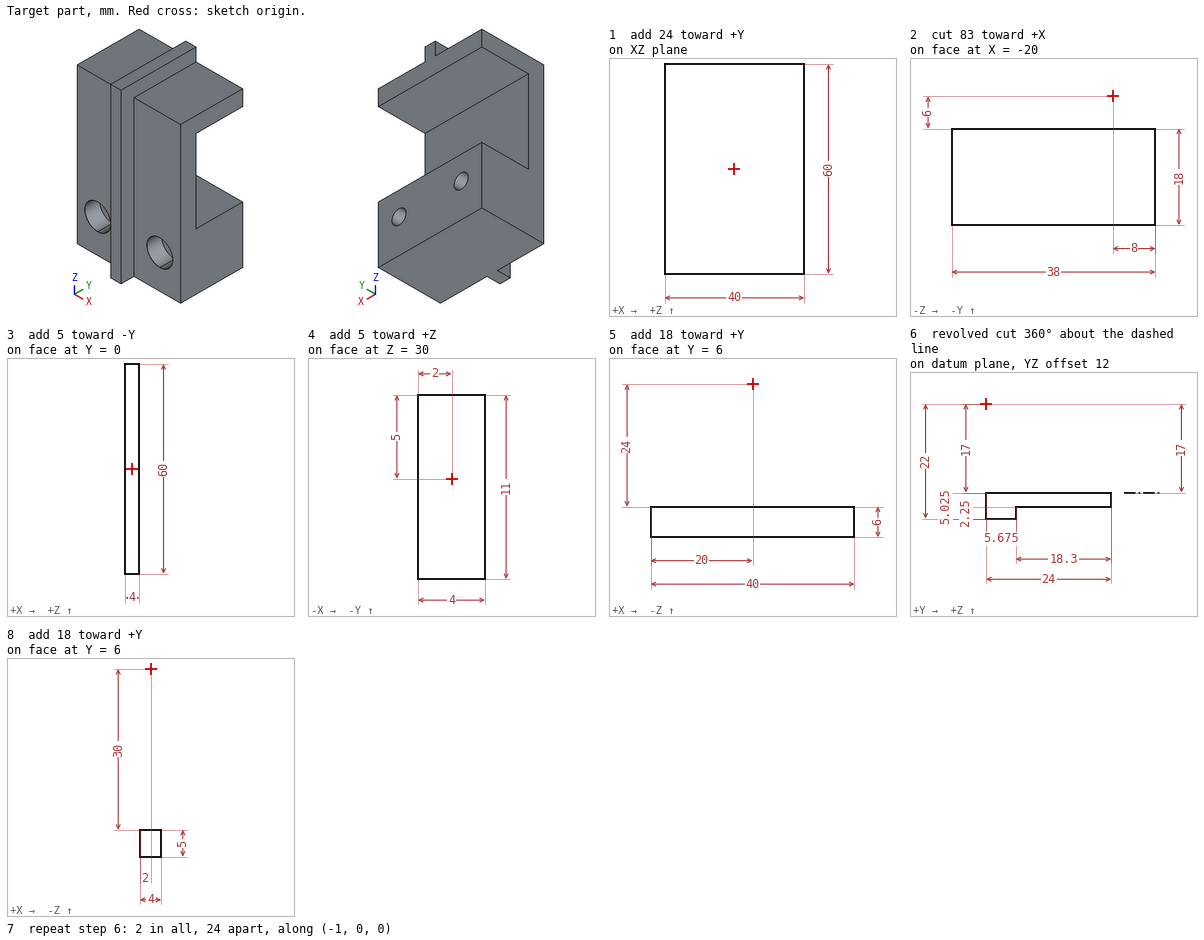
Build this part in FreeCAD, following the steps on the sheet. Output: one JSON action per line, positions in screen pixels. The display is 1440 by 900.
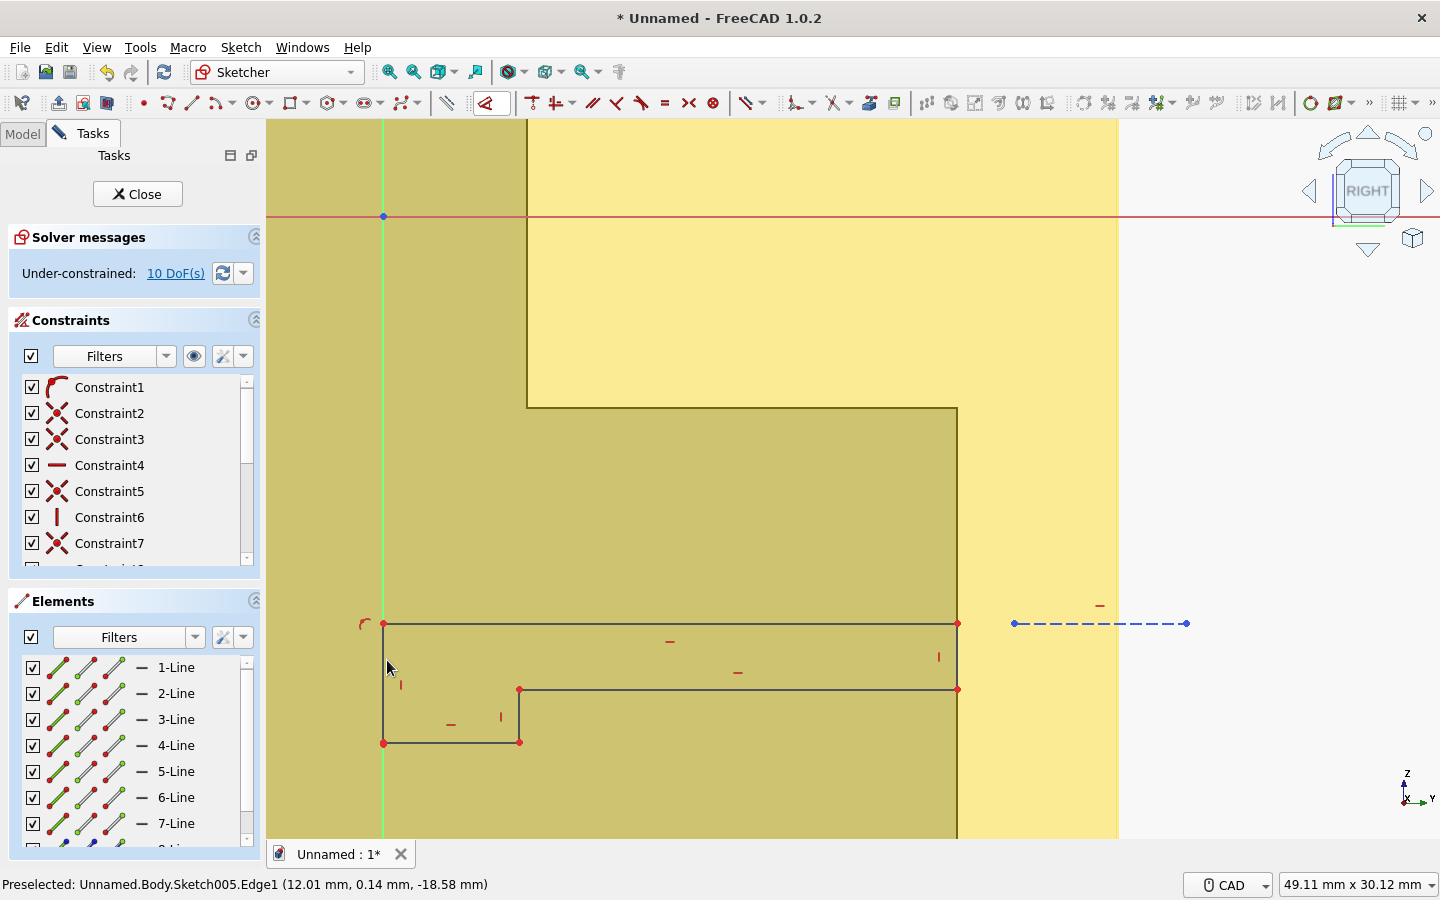
{"action": "key", "text": "d"}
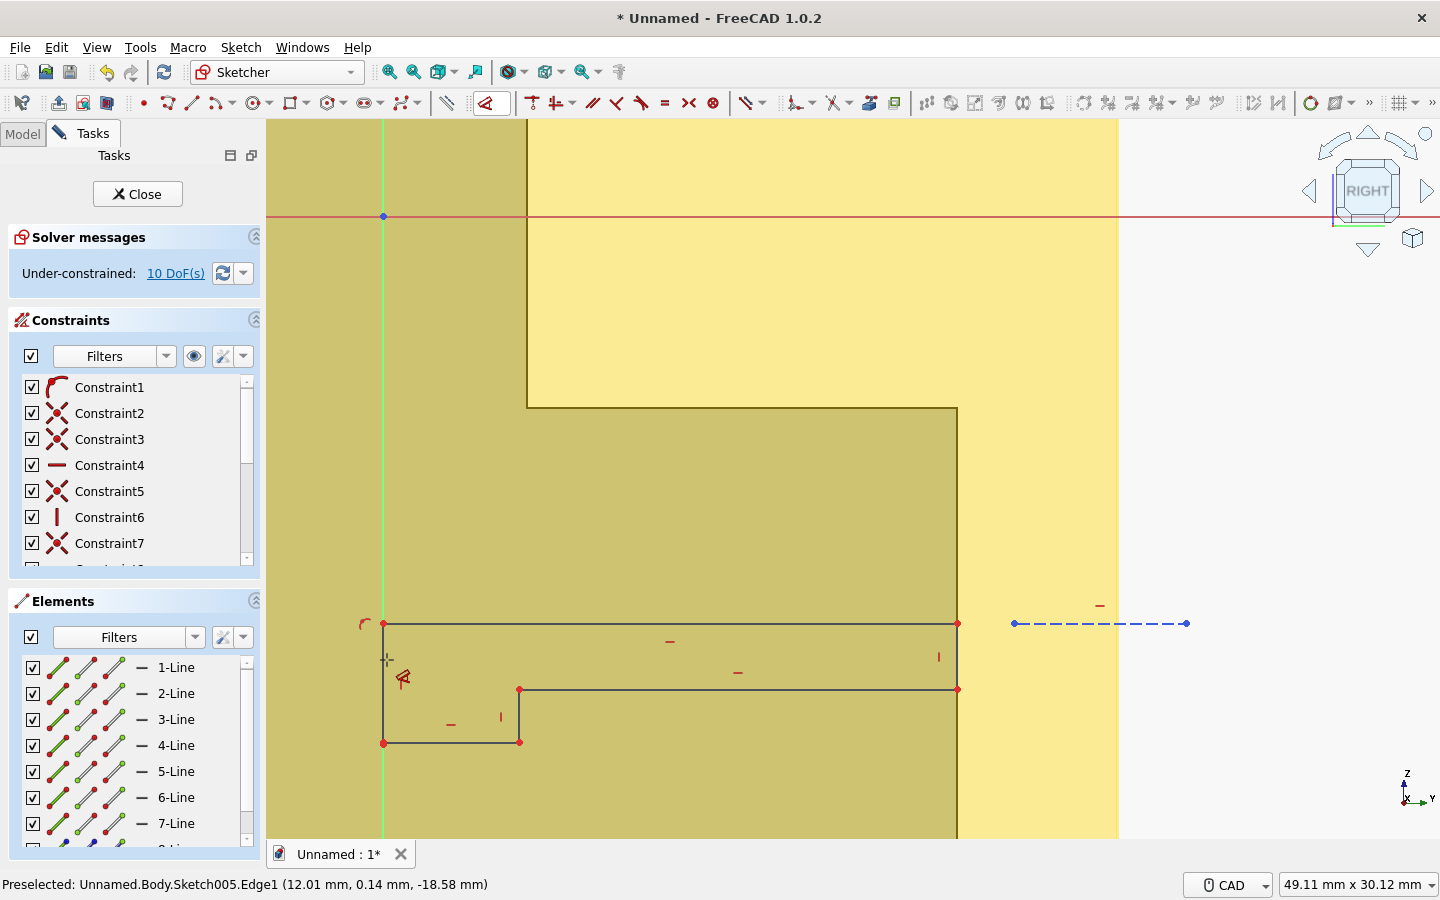
{"action": "left_click", "coordinate": [785, 624]}
{"action": "left_click", "coordinate": [670, 658]}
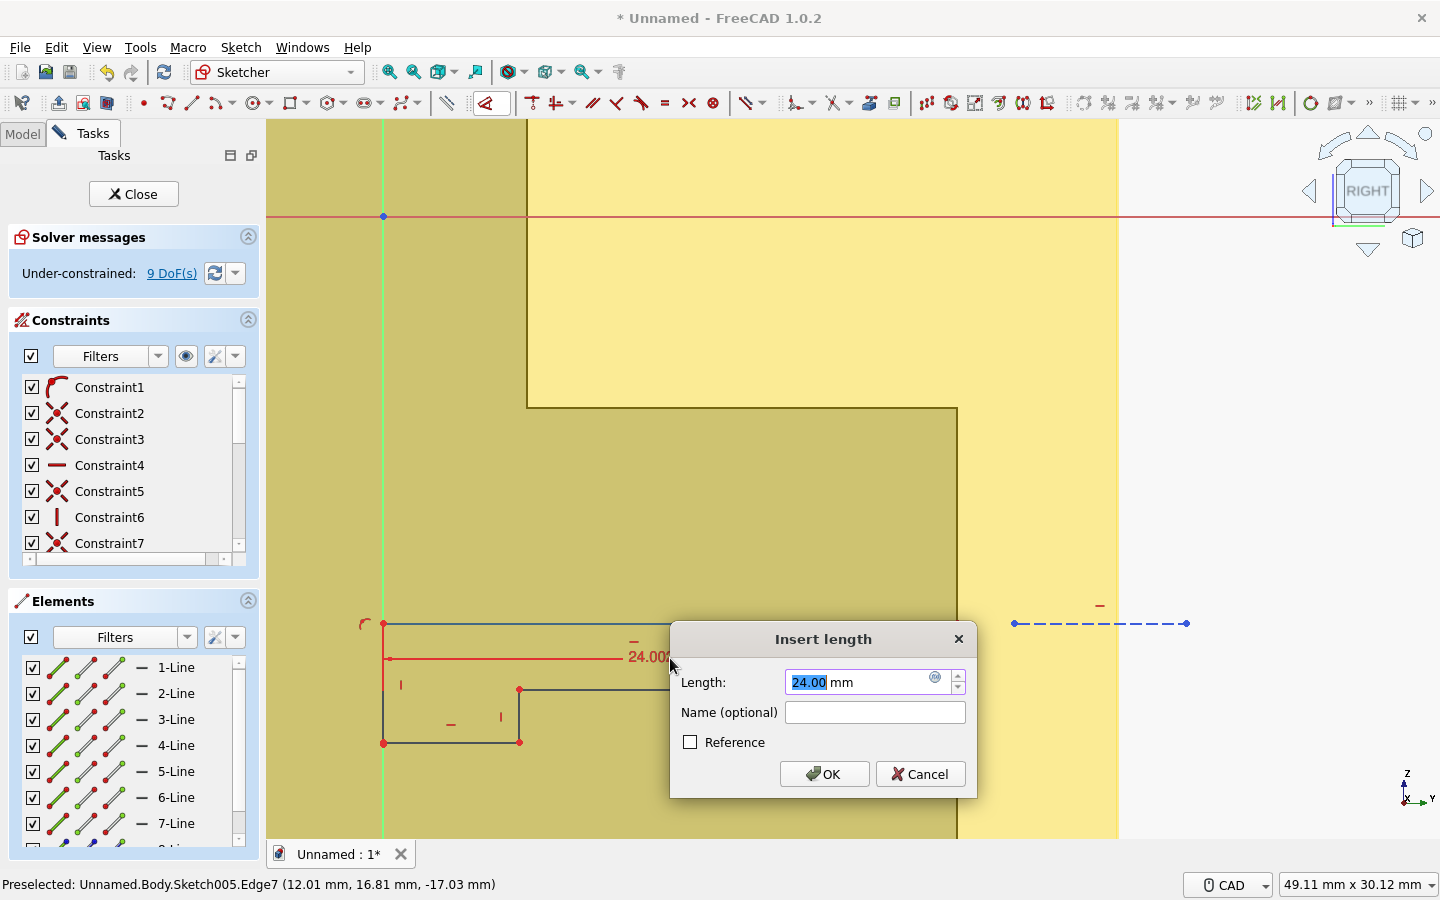
{"action": "type", "text": "24"}
{"action": "key", "text": "Return"}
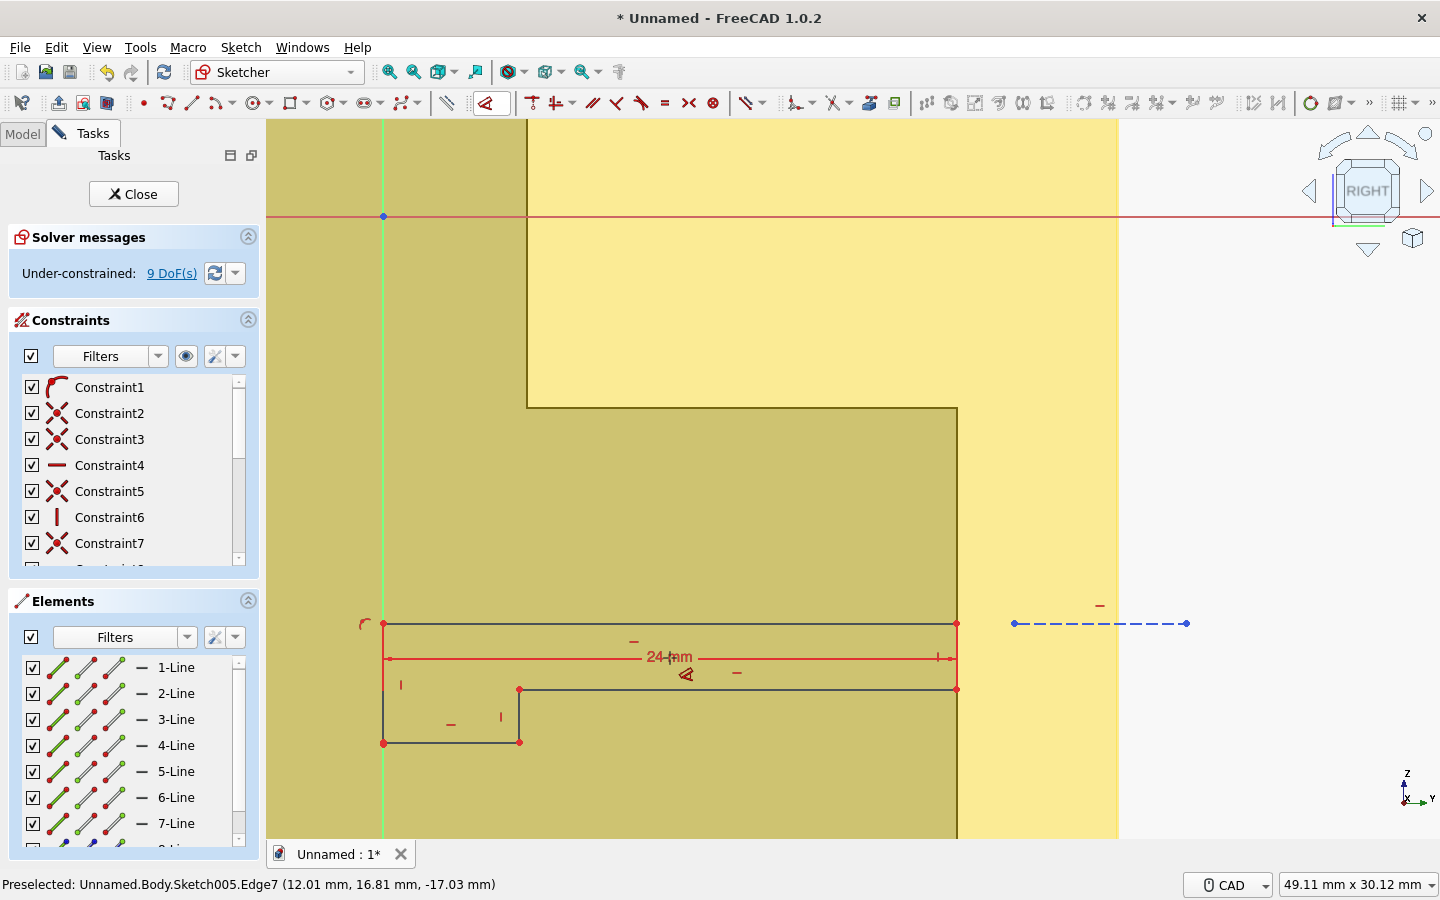
{"action": "left_click", "coordinate": [383, 624]}
{"action": "left_click", "coordinate": [349, 420]}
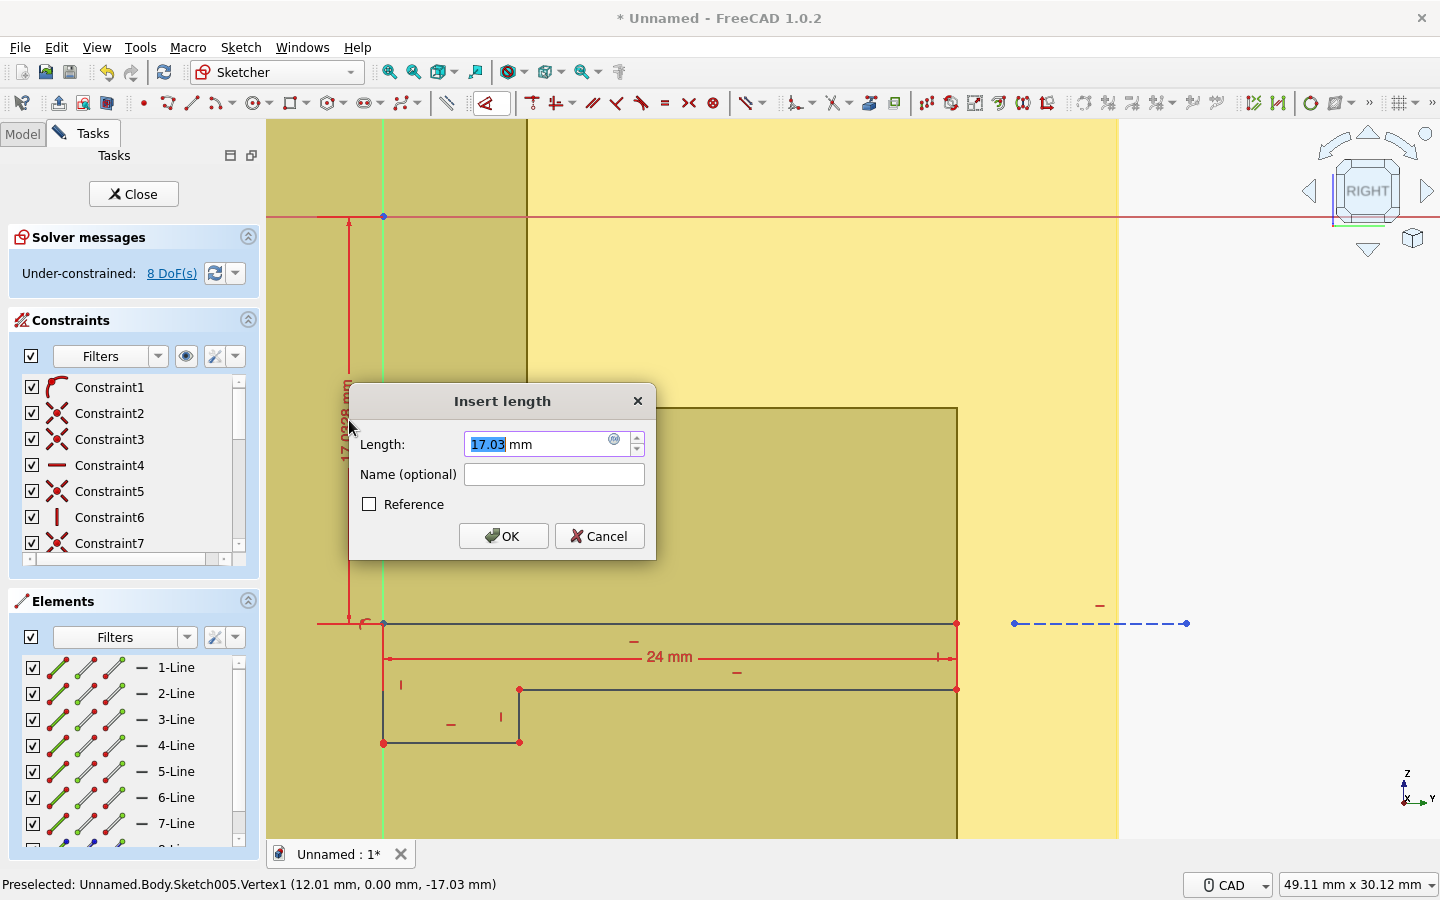
{"action": "type", "text": "17"}
{"action": "key", "text": "Return"}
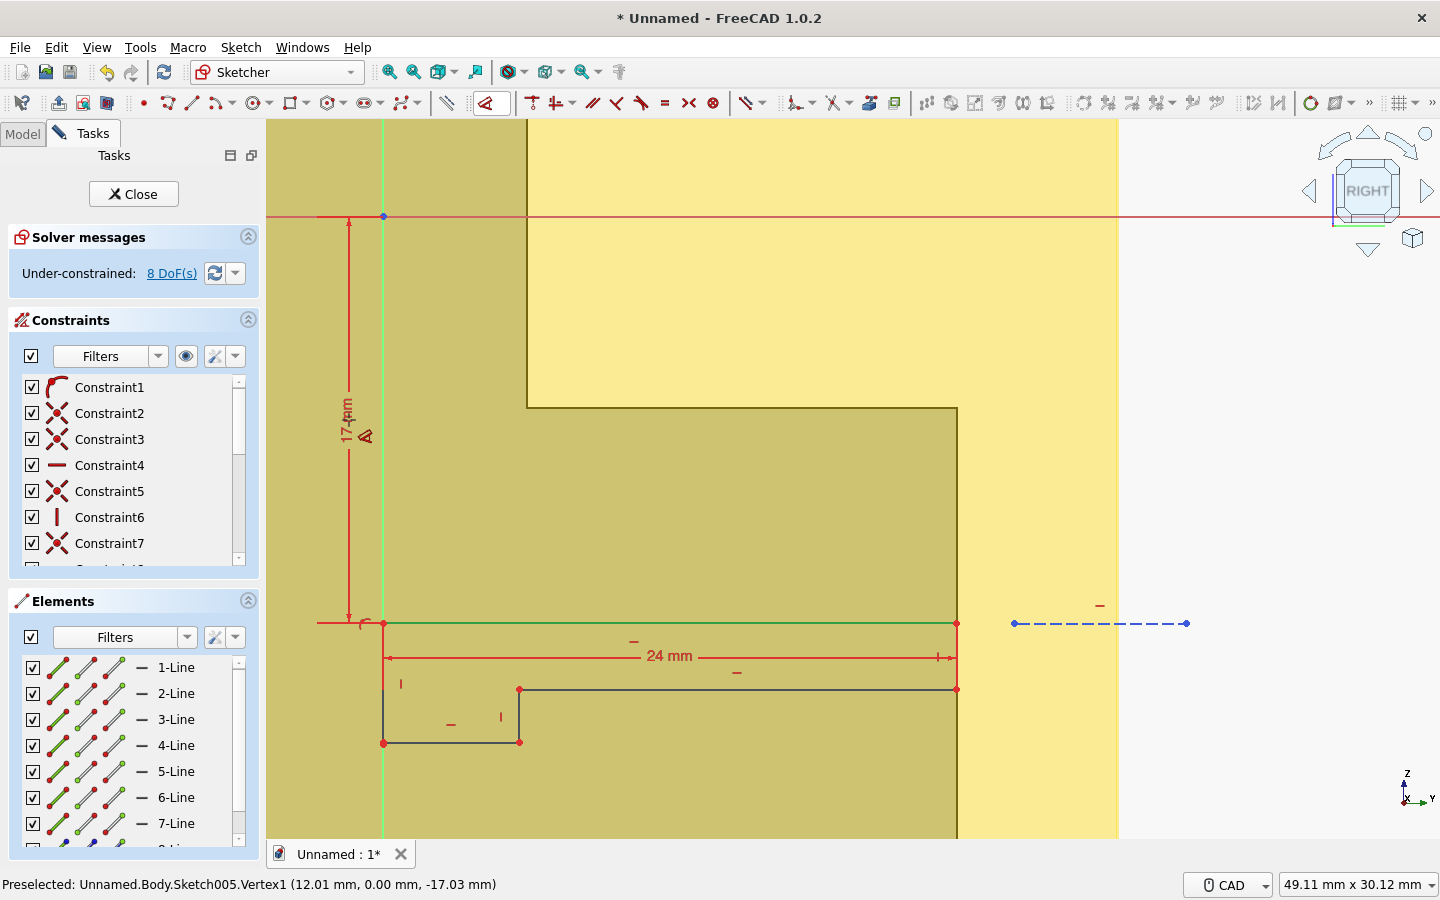
{"action": "scroll", "coordinate": [384, 743], "scroll_direction": "up", "scroll_amount": 10}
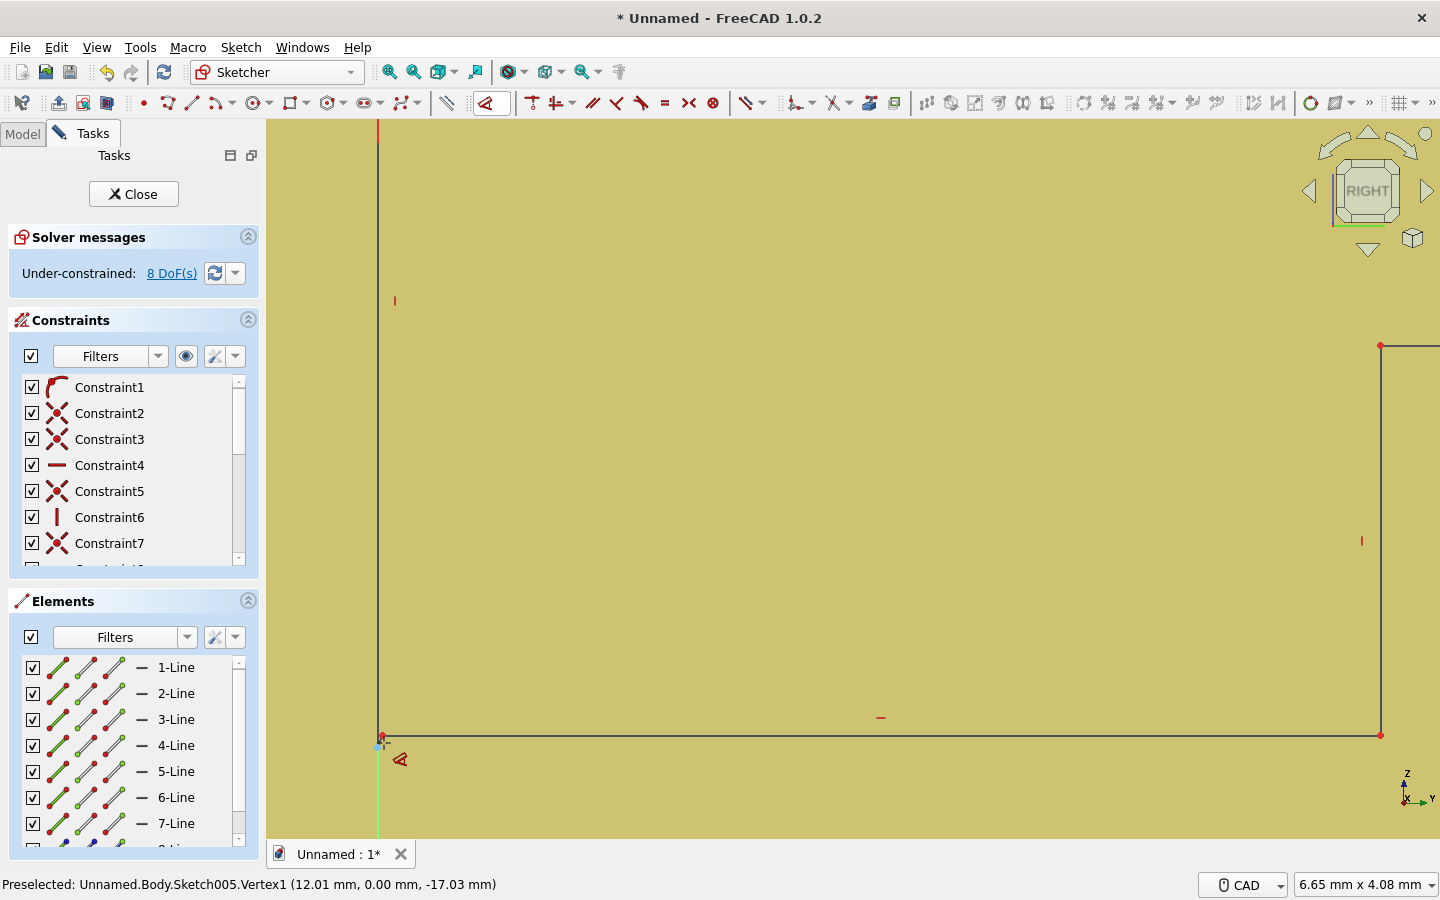
{"action": "left_click", "coordinate": [382, 736]}
{"action": "left_click", "coordinate": [344, 441]}